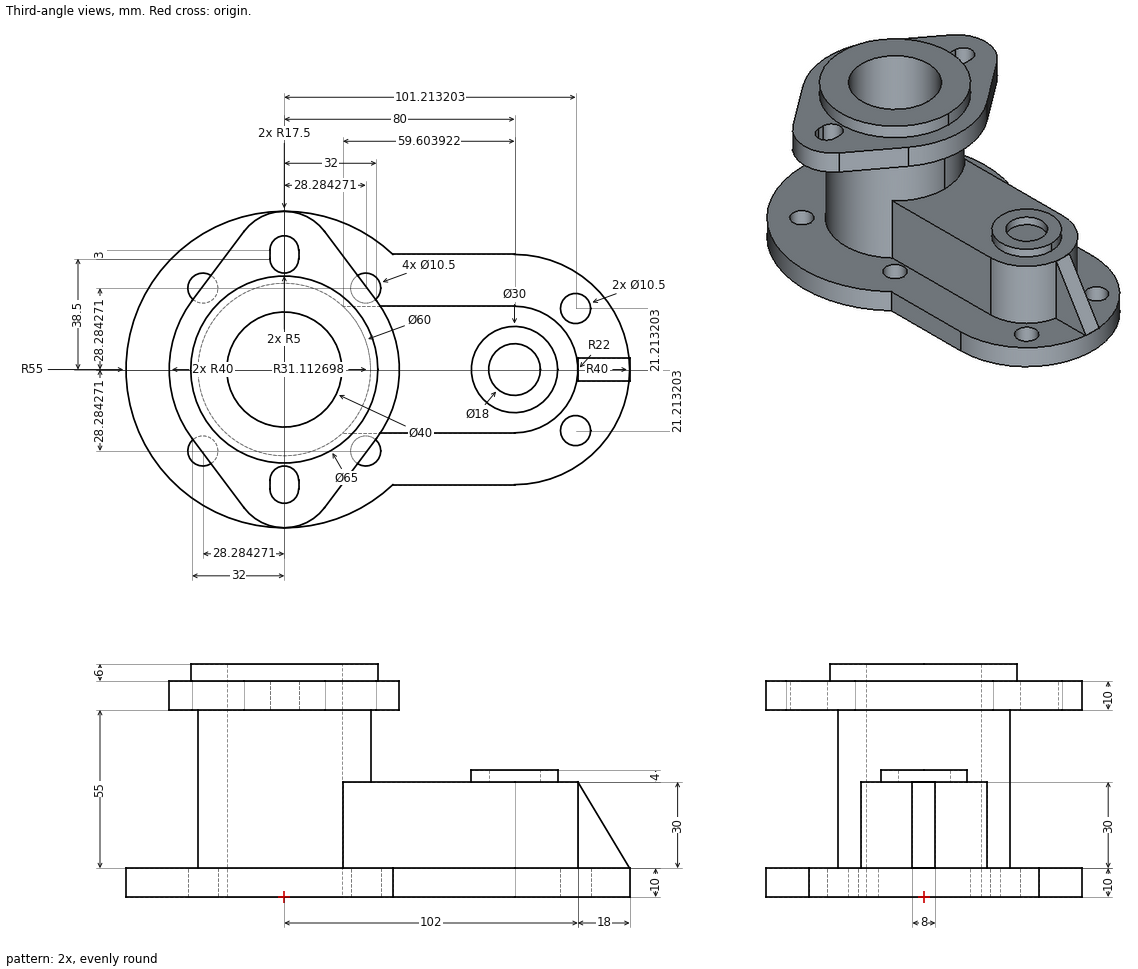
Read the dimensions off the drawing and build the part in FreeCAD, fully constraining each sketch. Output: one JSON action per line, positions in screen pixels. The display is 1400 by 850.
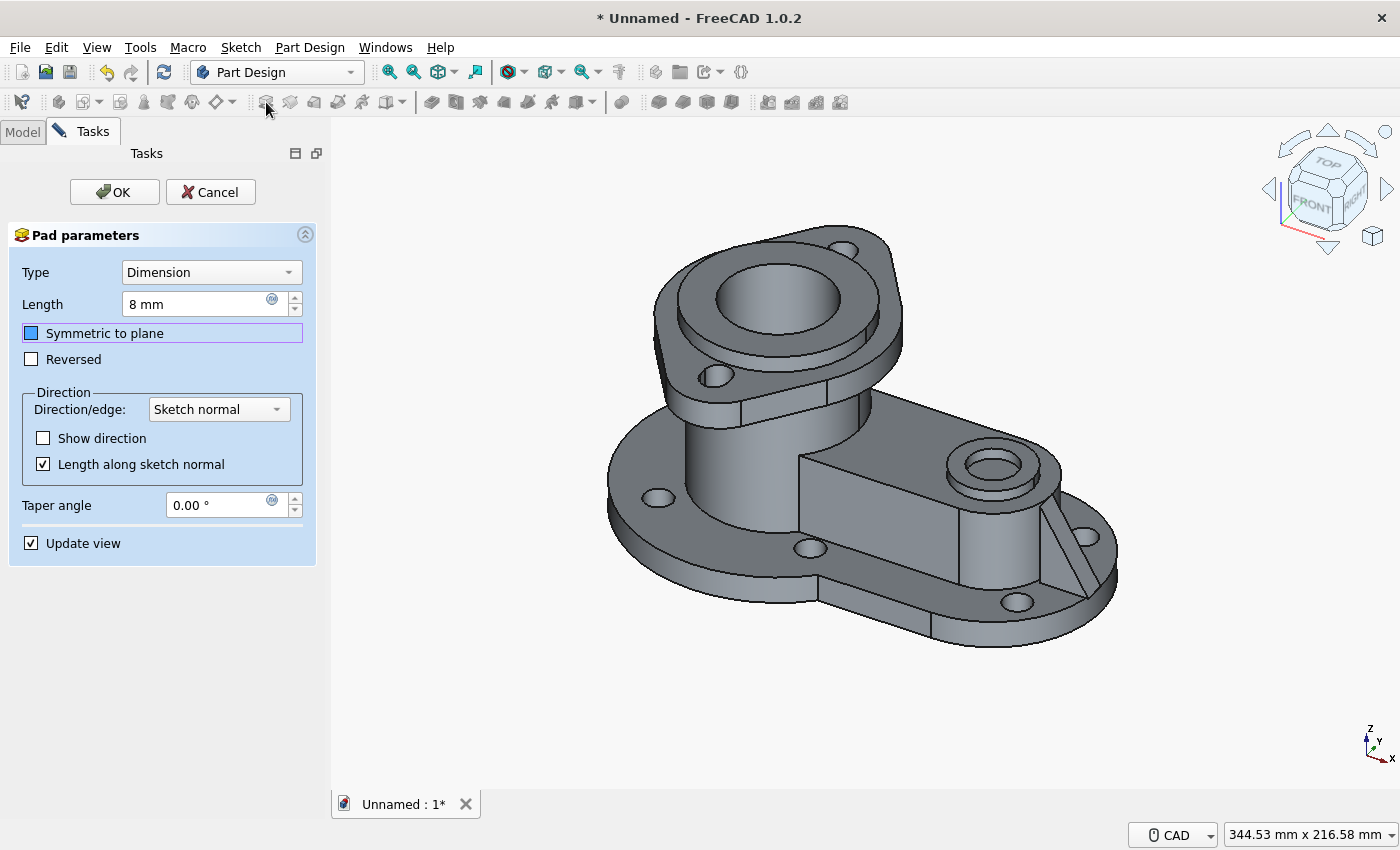
{"action": "left_click", "coordinate": [30, 333]}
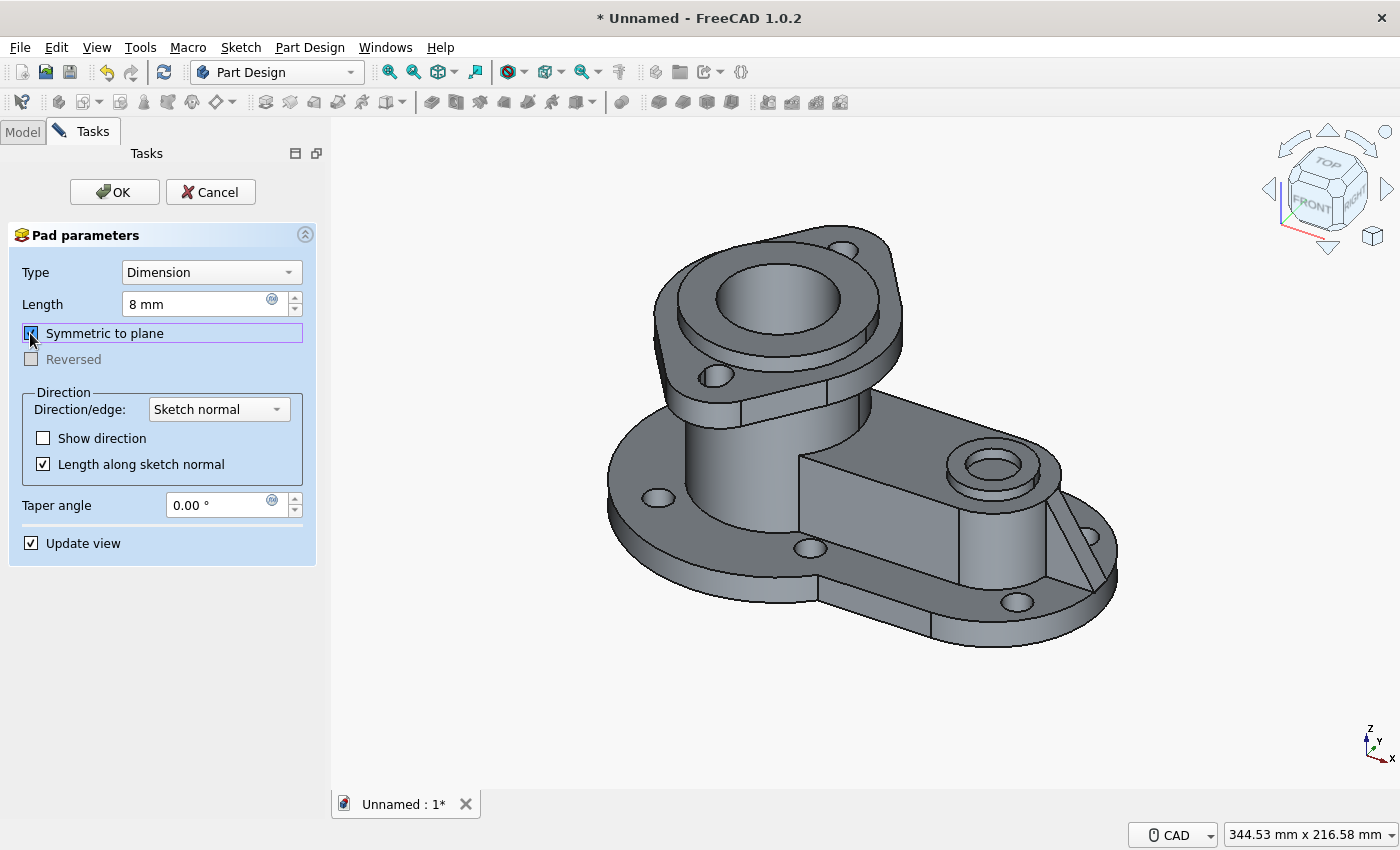
{"action": "left_click", "coordinate": [115, 192]}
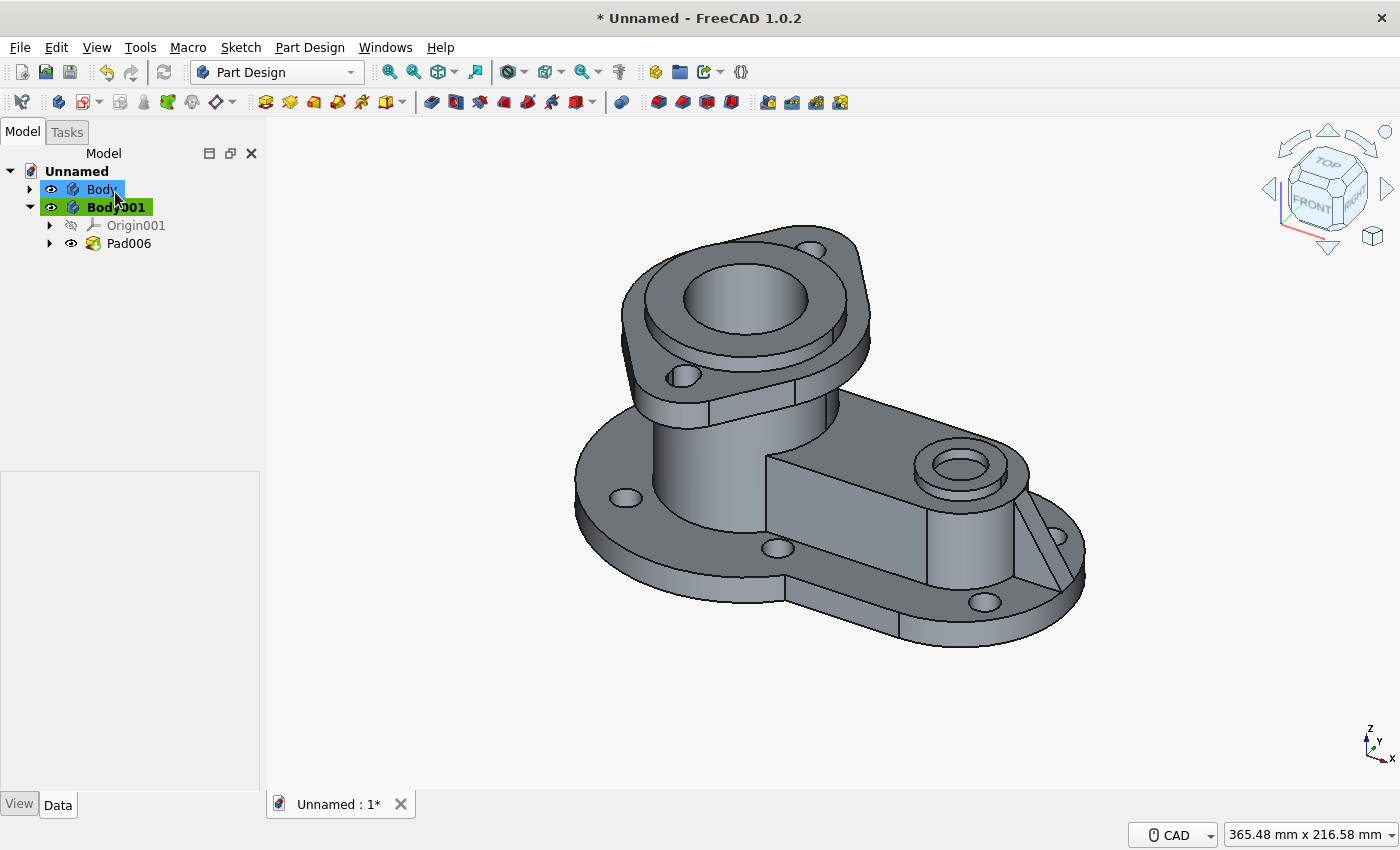
{"action": "key", "text": "0"}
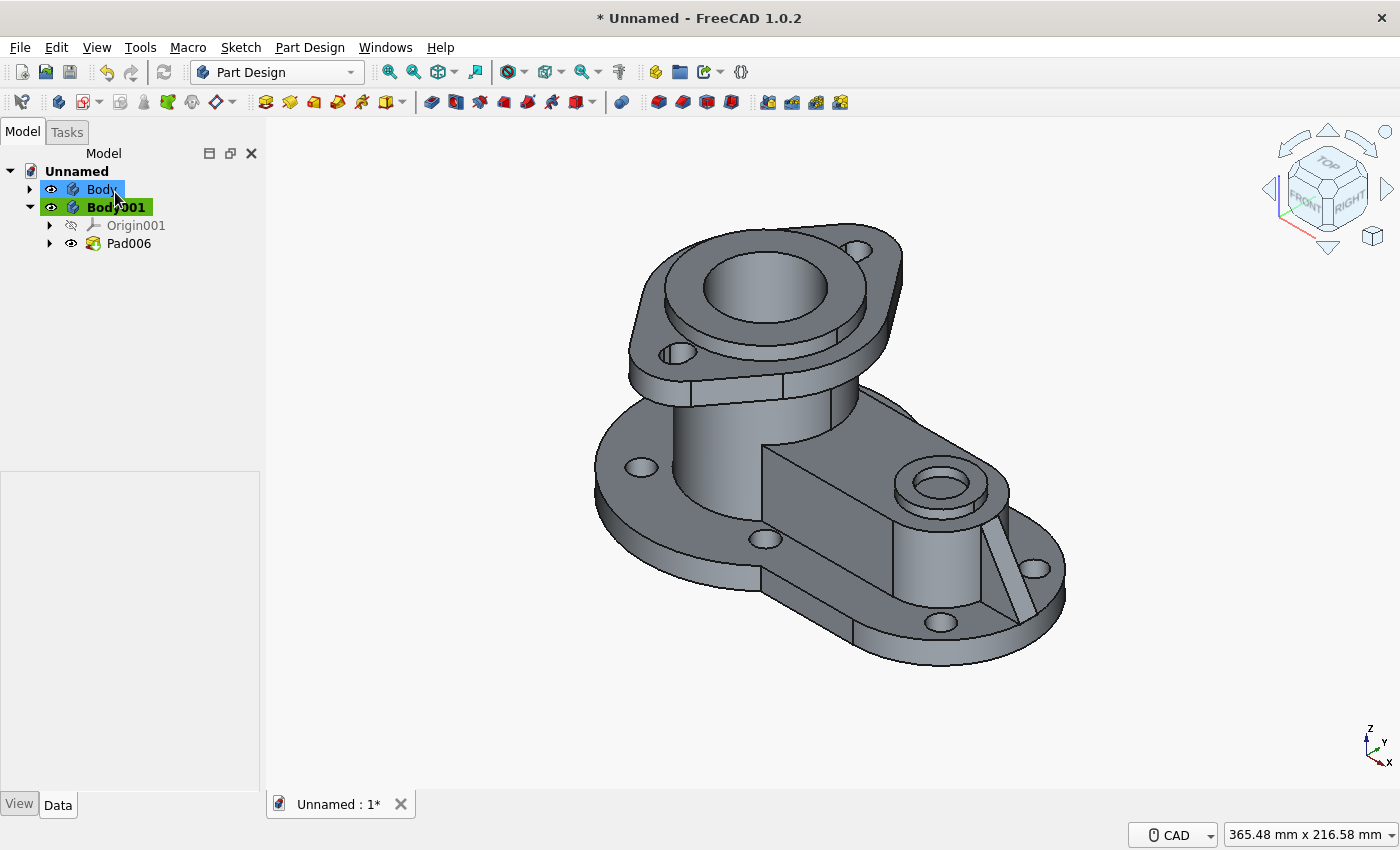
{"action": "key", "text": "v f"}